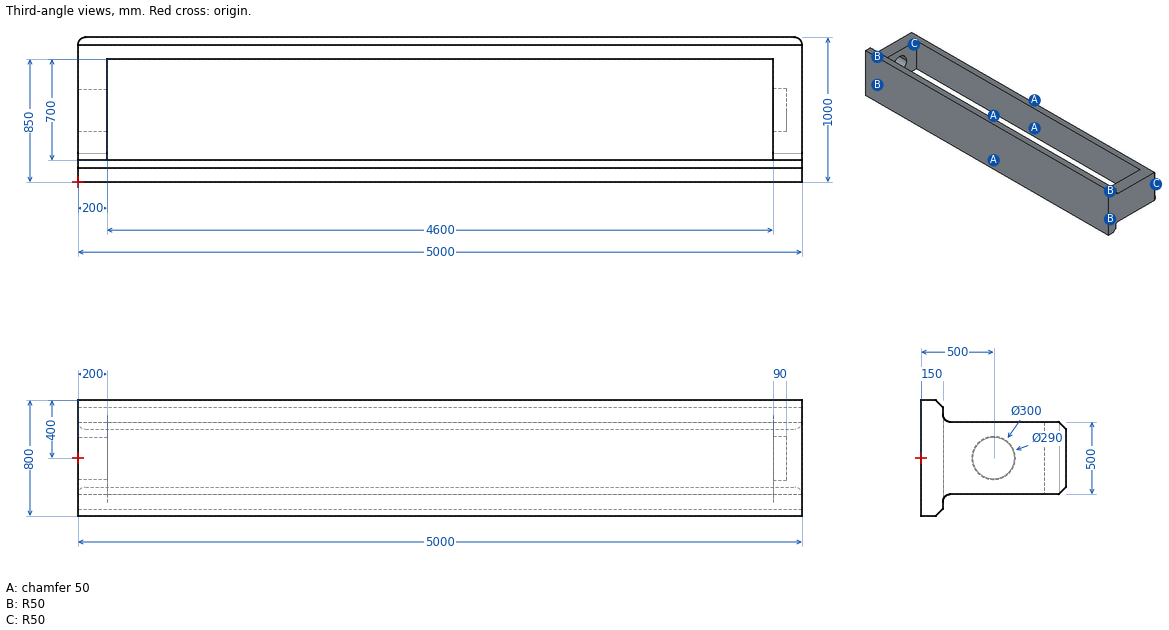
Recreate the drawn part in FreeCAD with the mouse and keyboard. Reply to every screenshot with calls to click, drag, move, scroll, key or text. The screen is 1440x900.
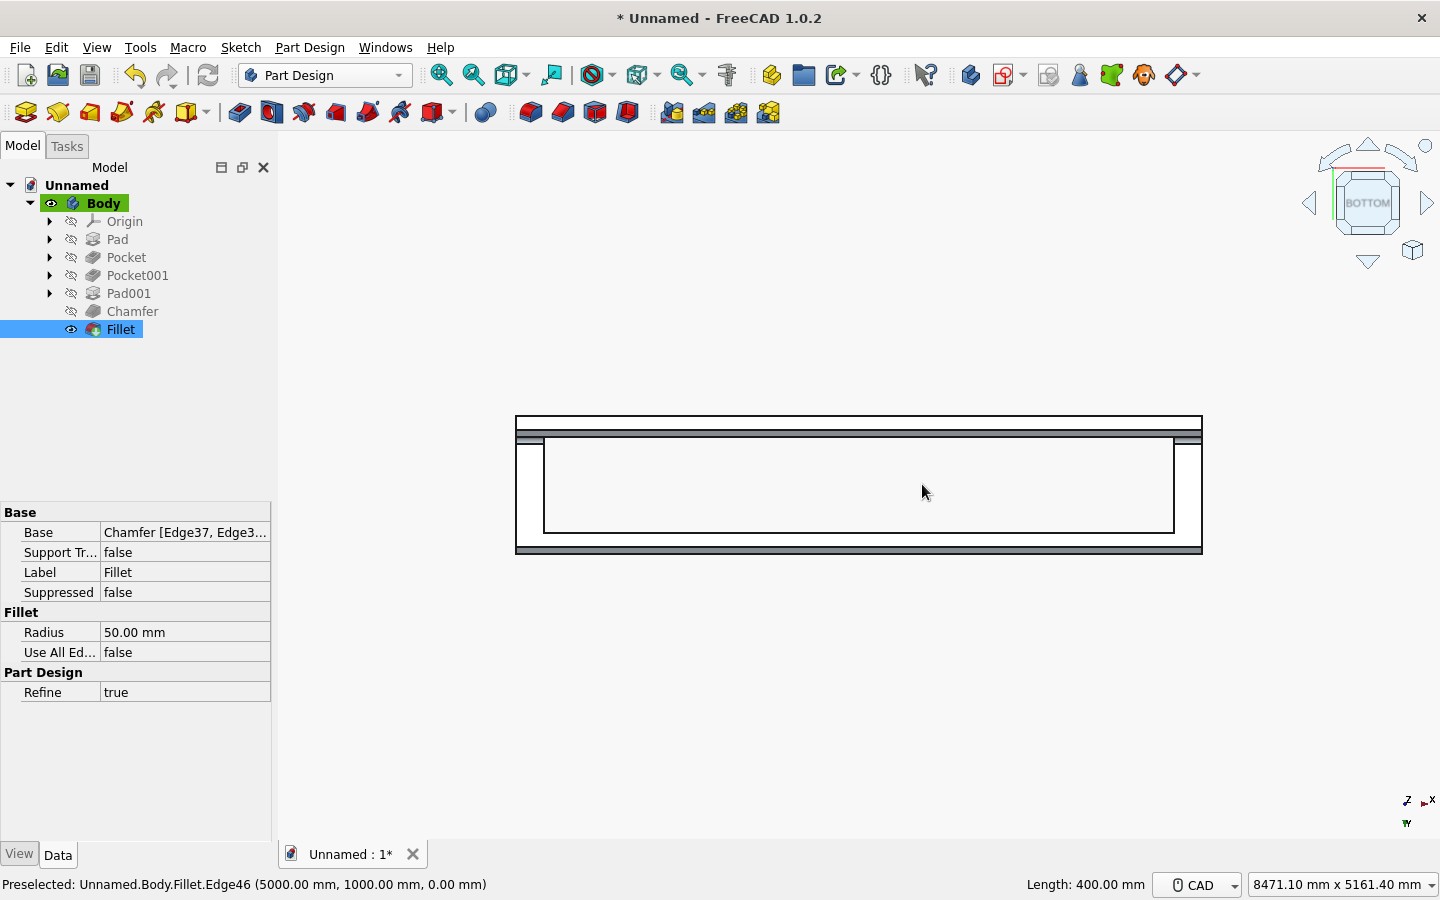
key(4)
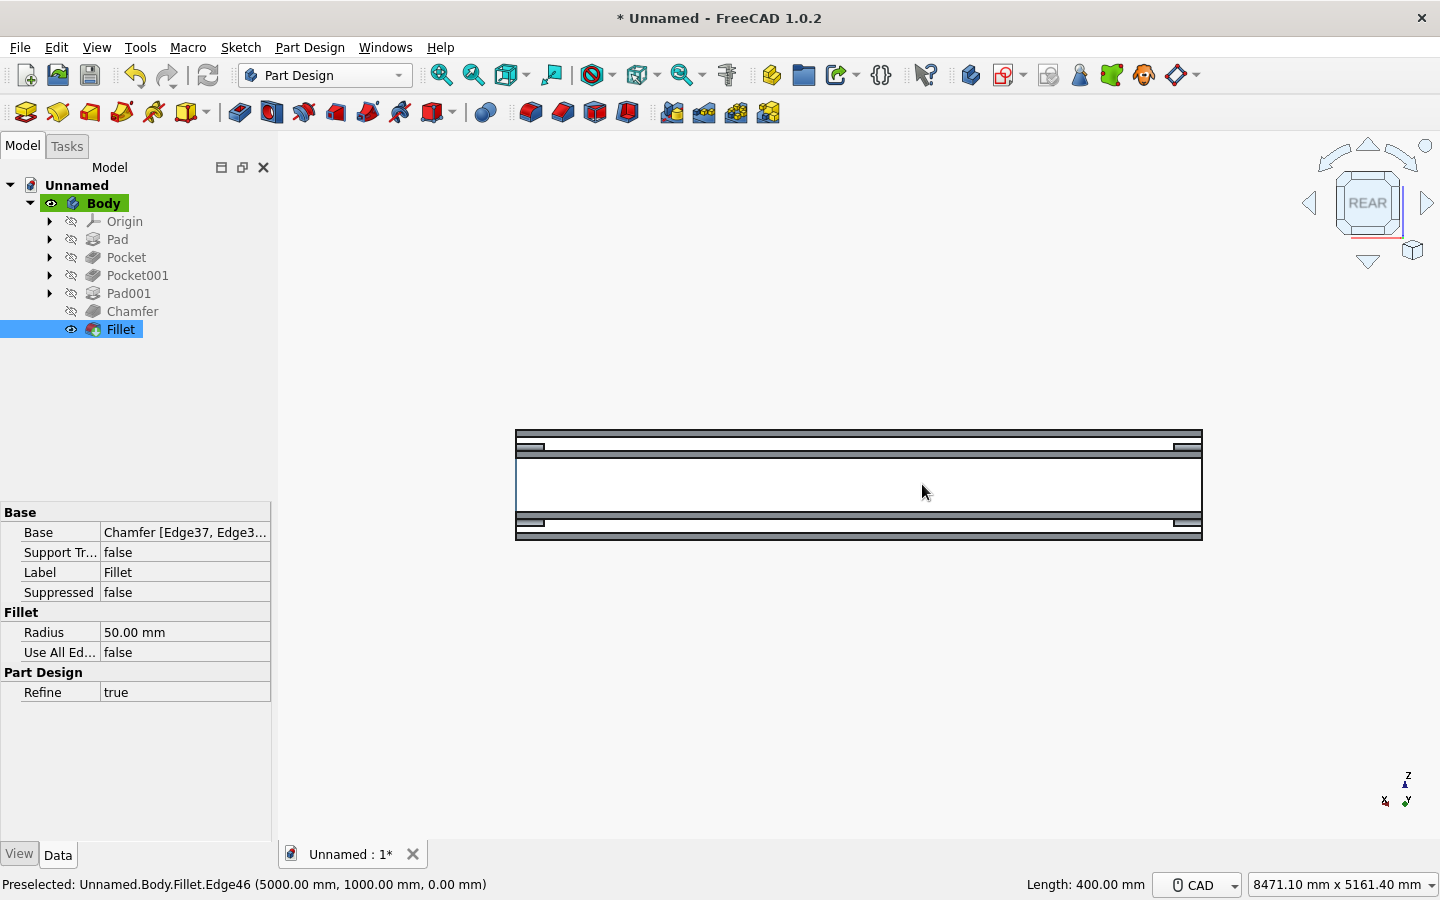
click(1202, 484, ctrl)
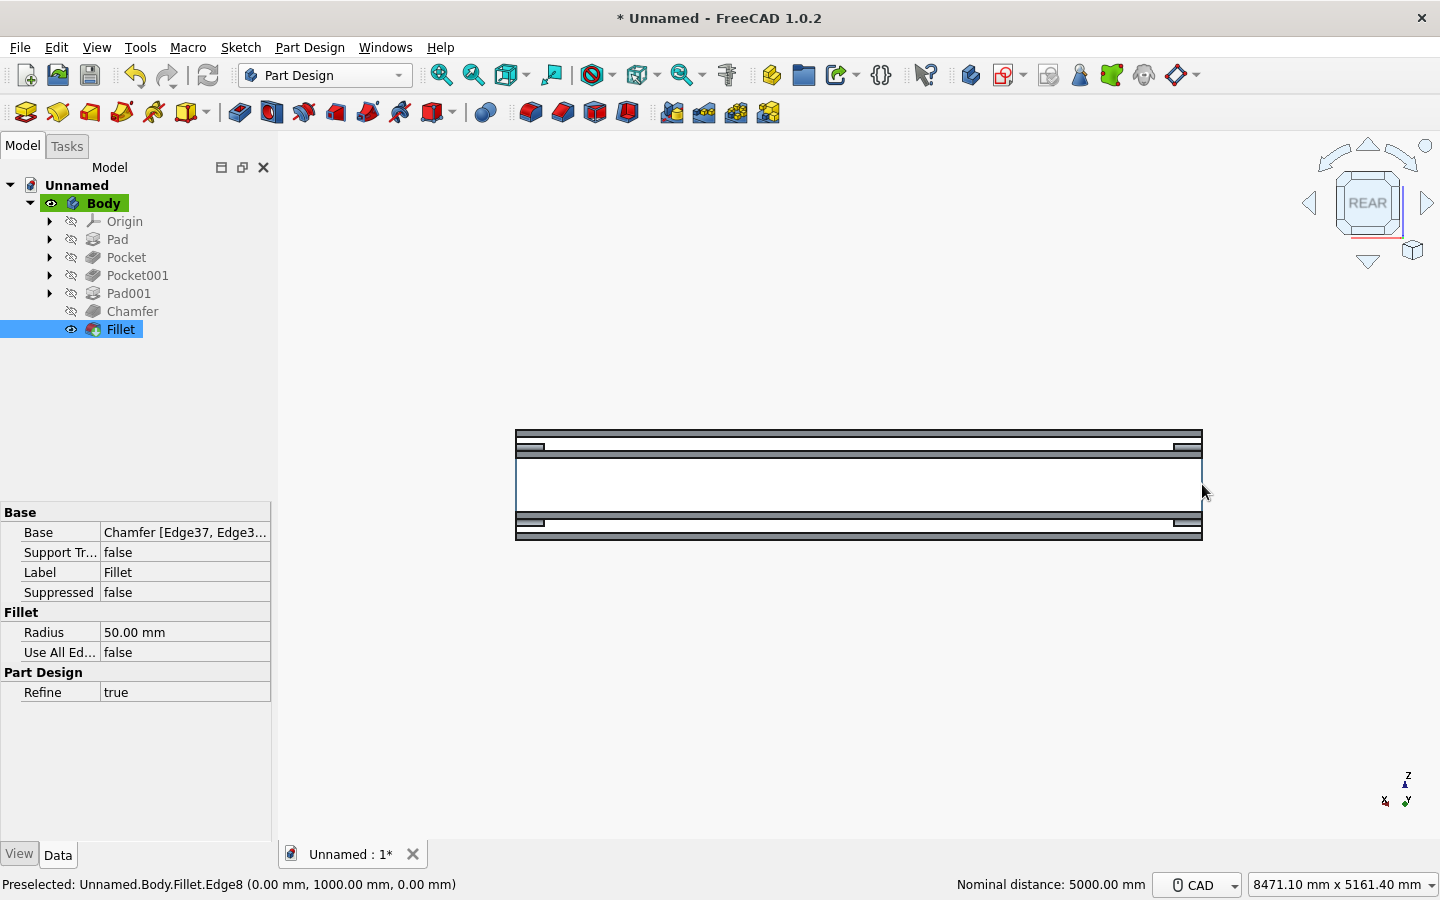
click(532, 112)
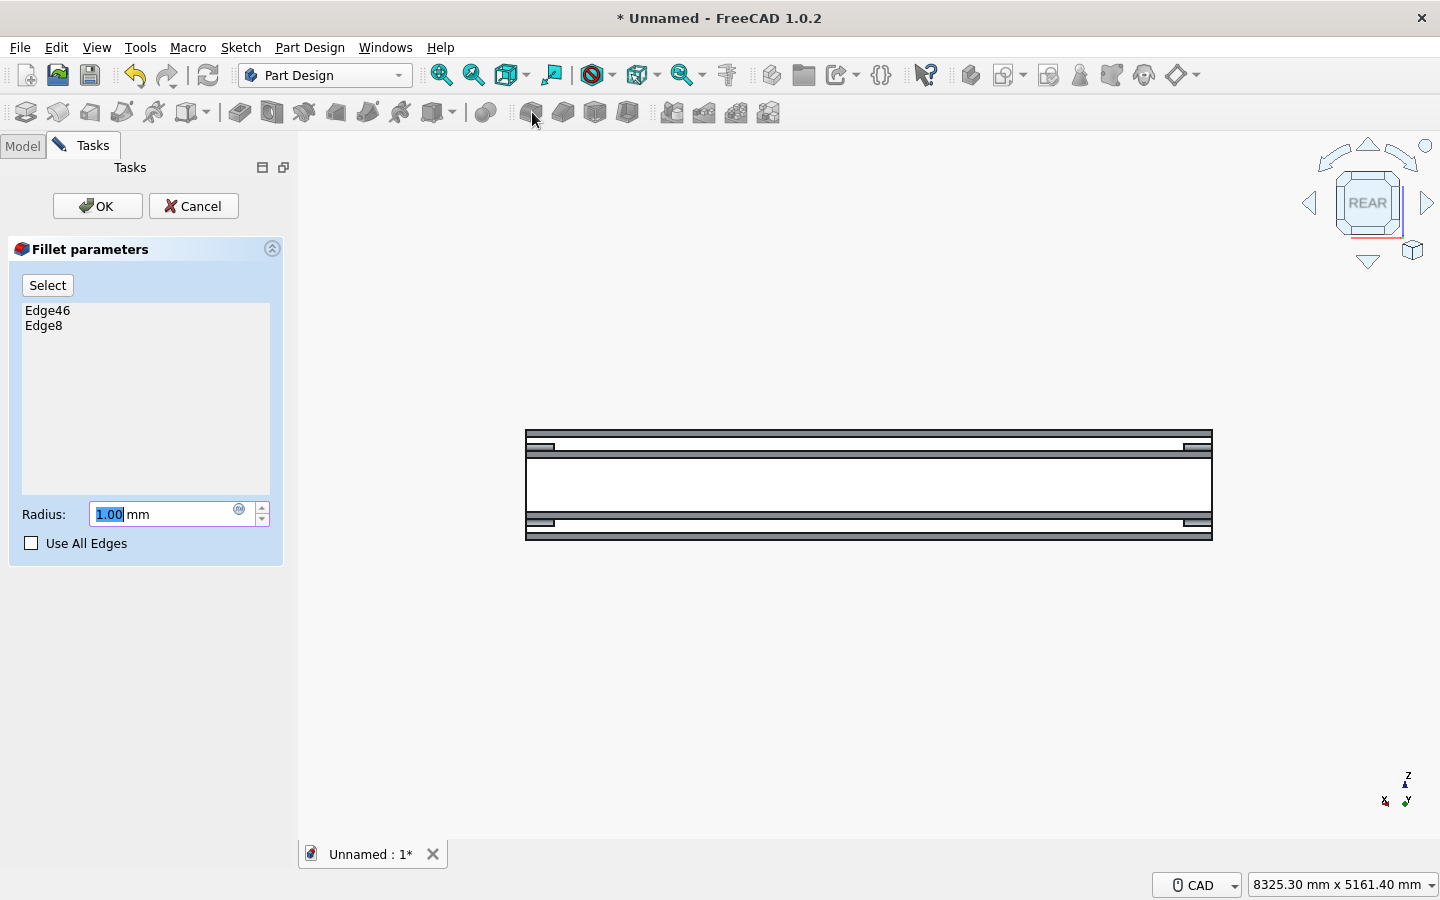
text(50)
key(Tab)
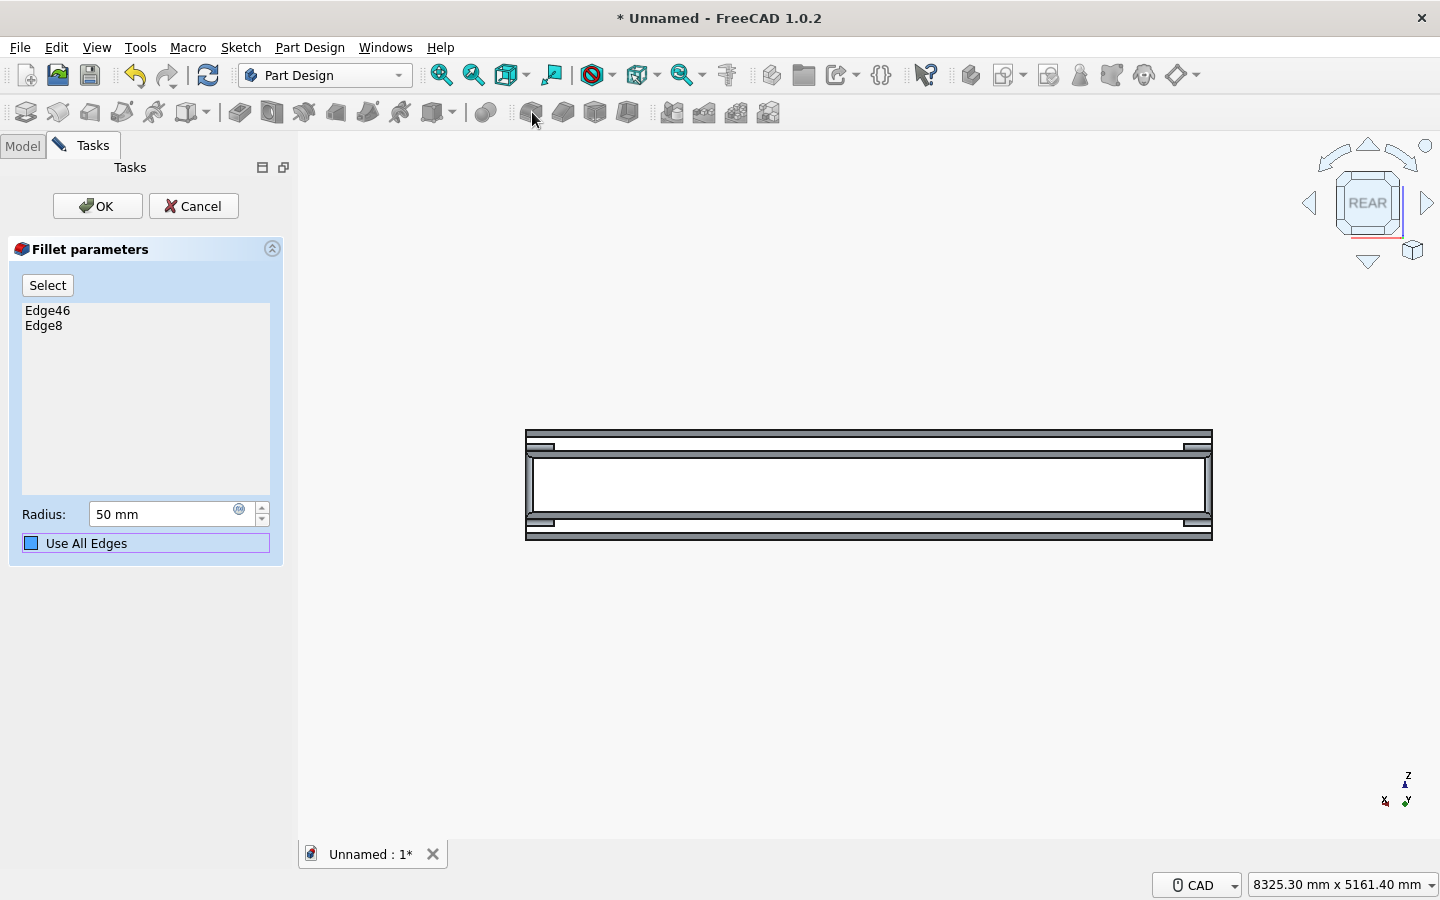
click(98, 206)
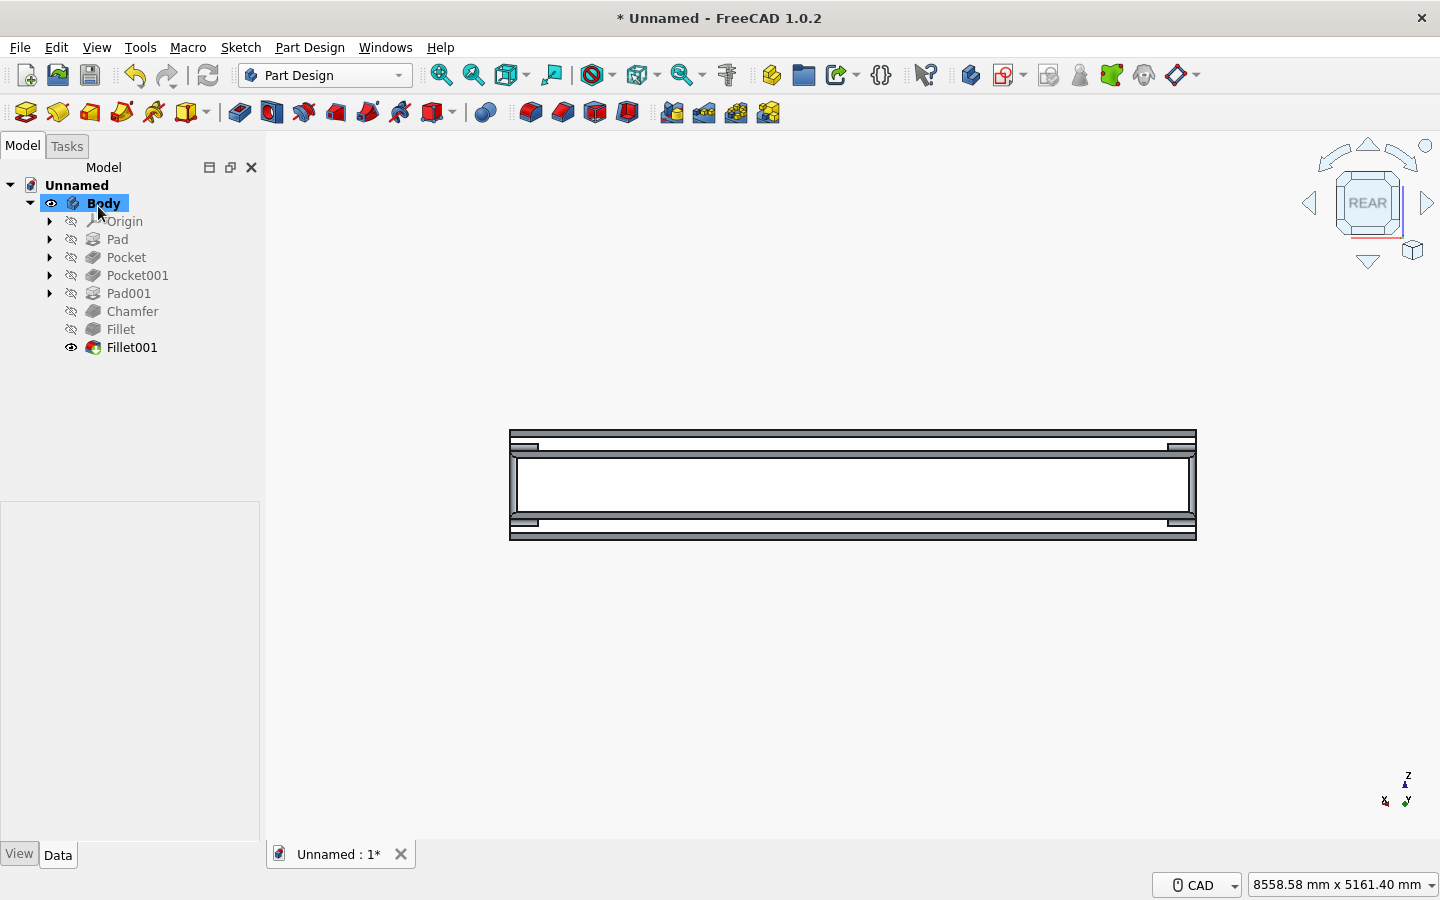
key(6)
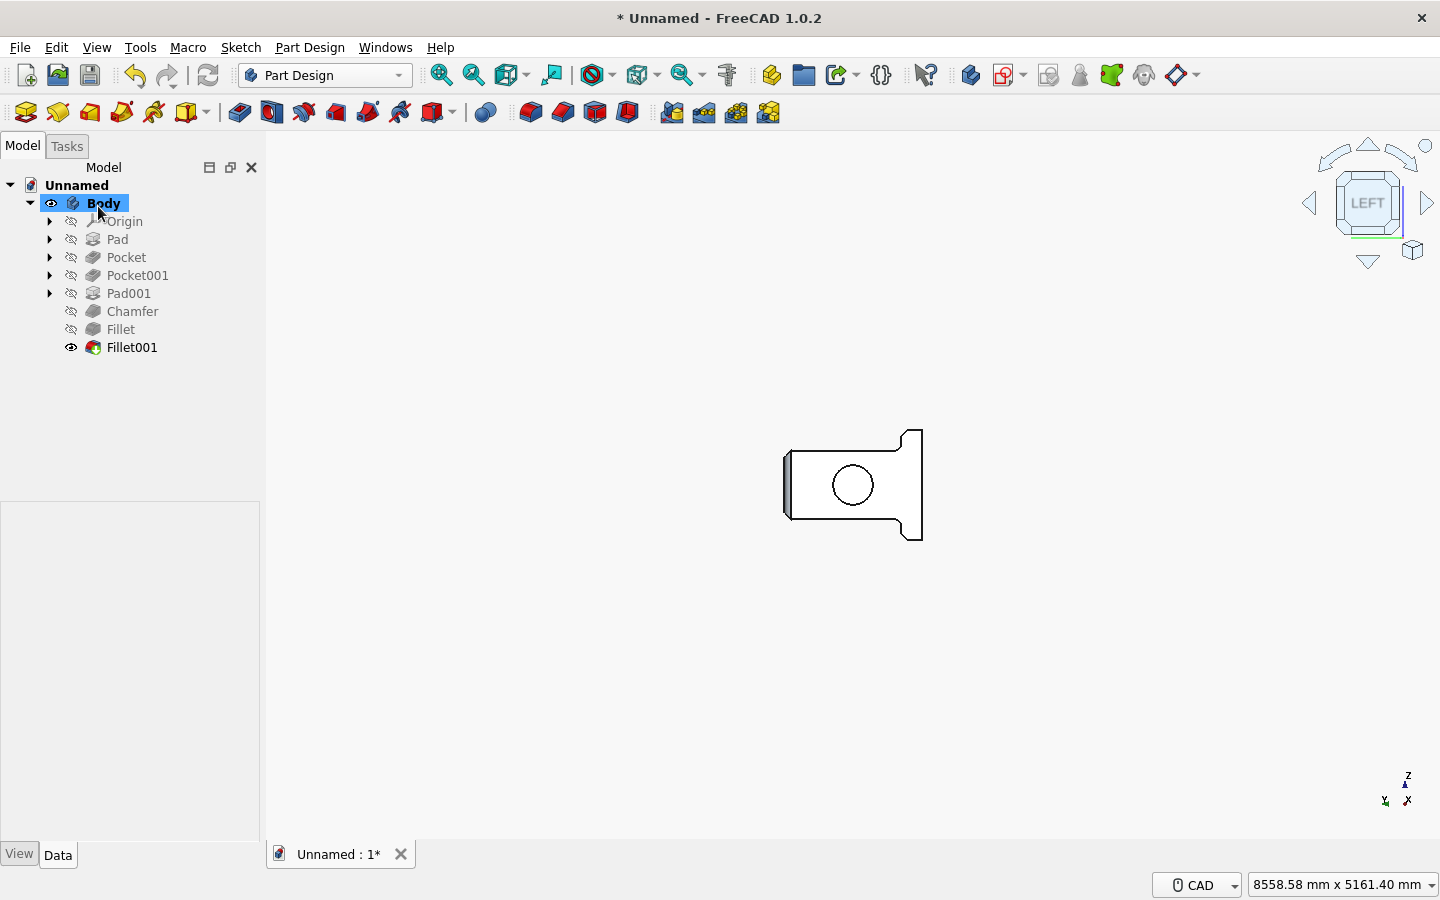
click(442, 76)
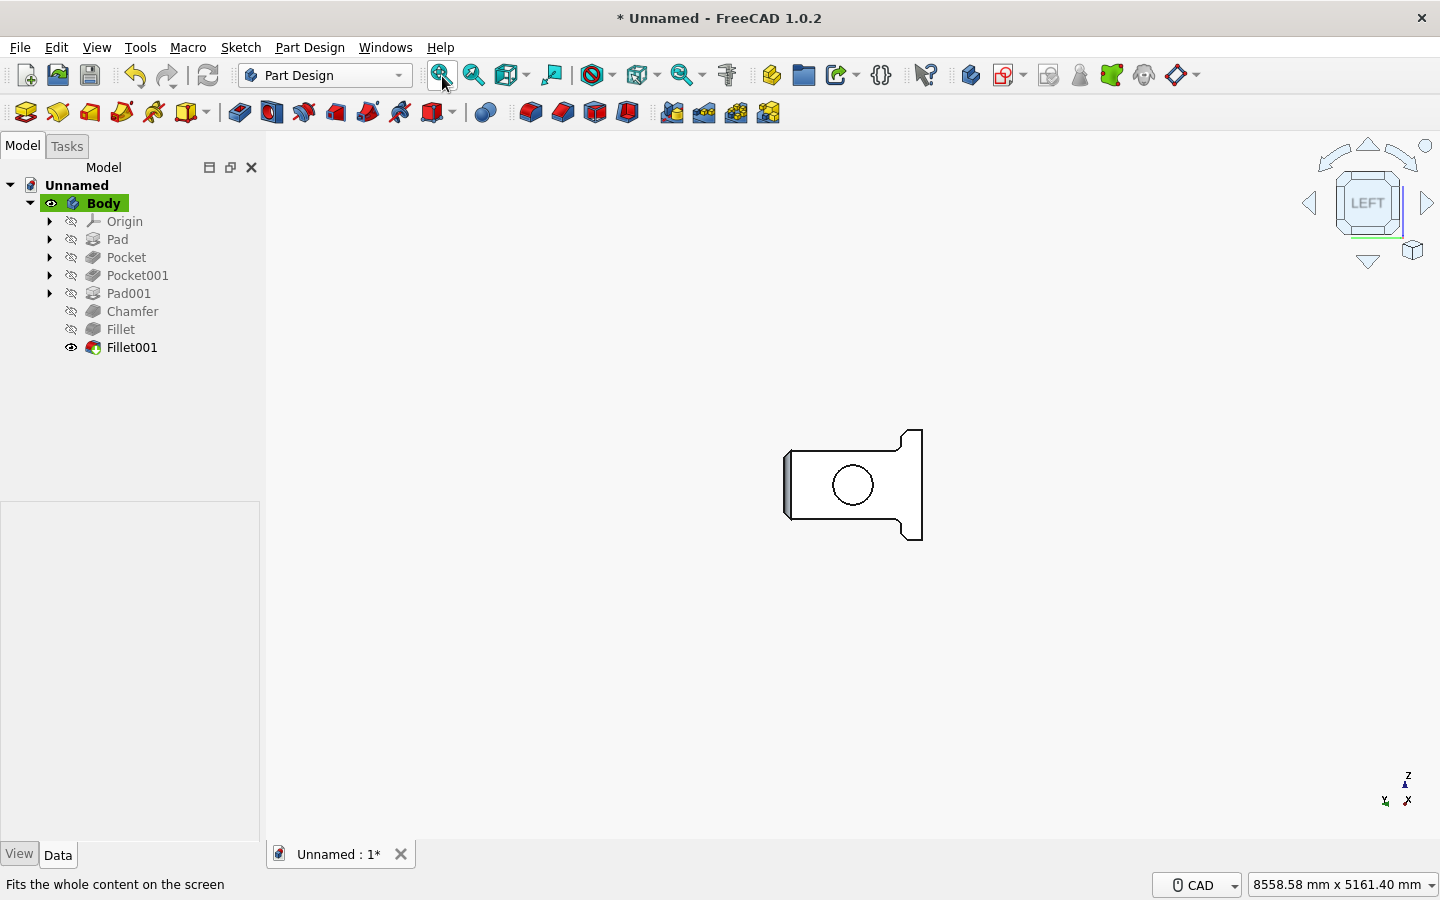
click(853, 484)